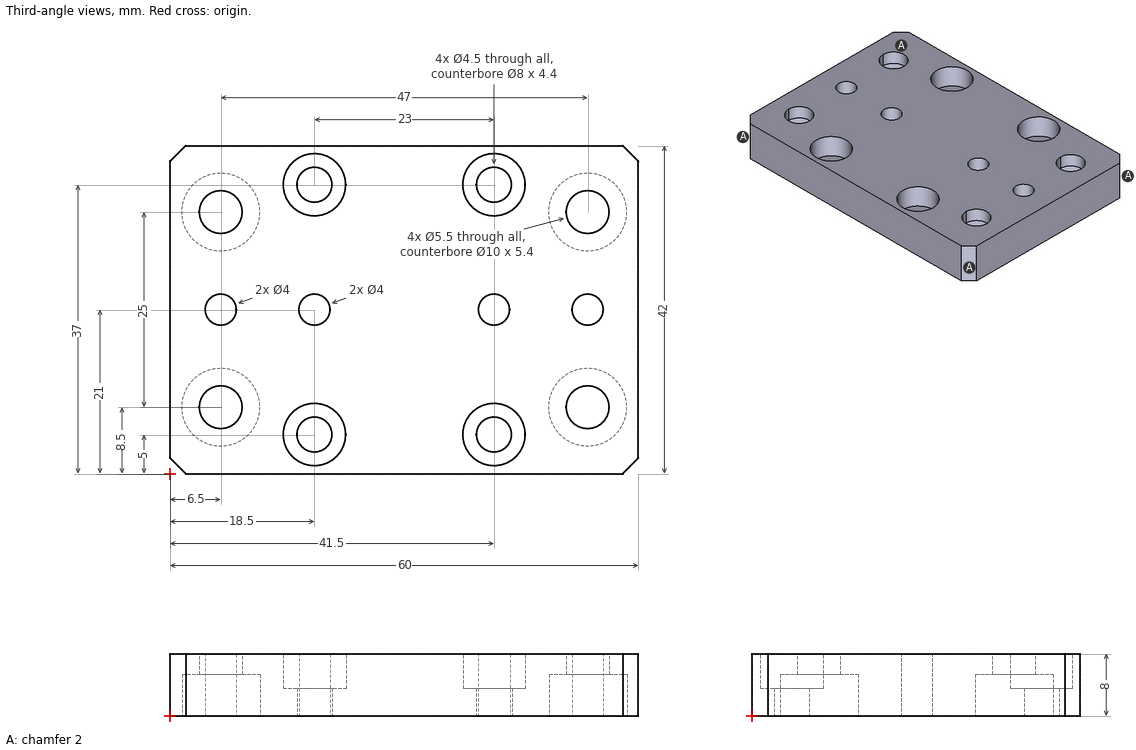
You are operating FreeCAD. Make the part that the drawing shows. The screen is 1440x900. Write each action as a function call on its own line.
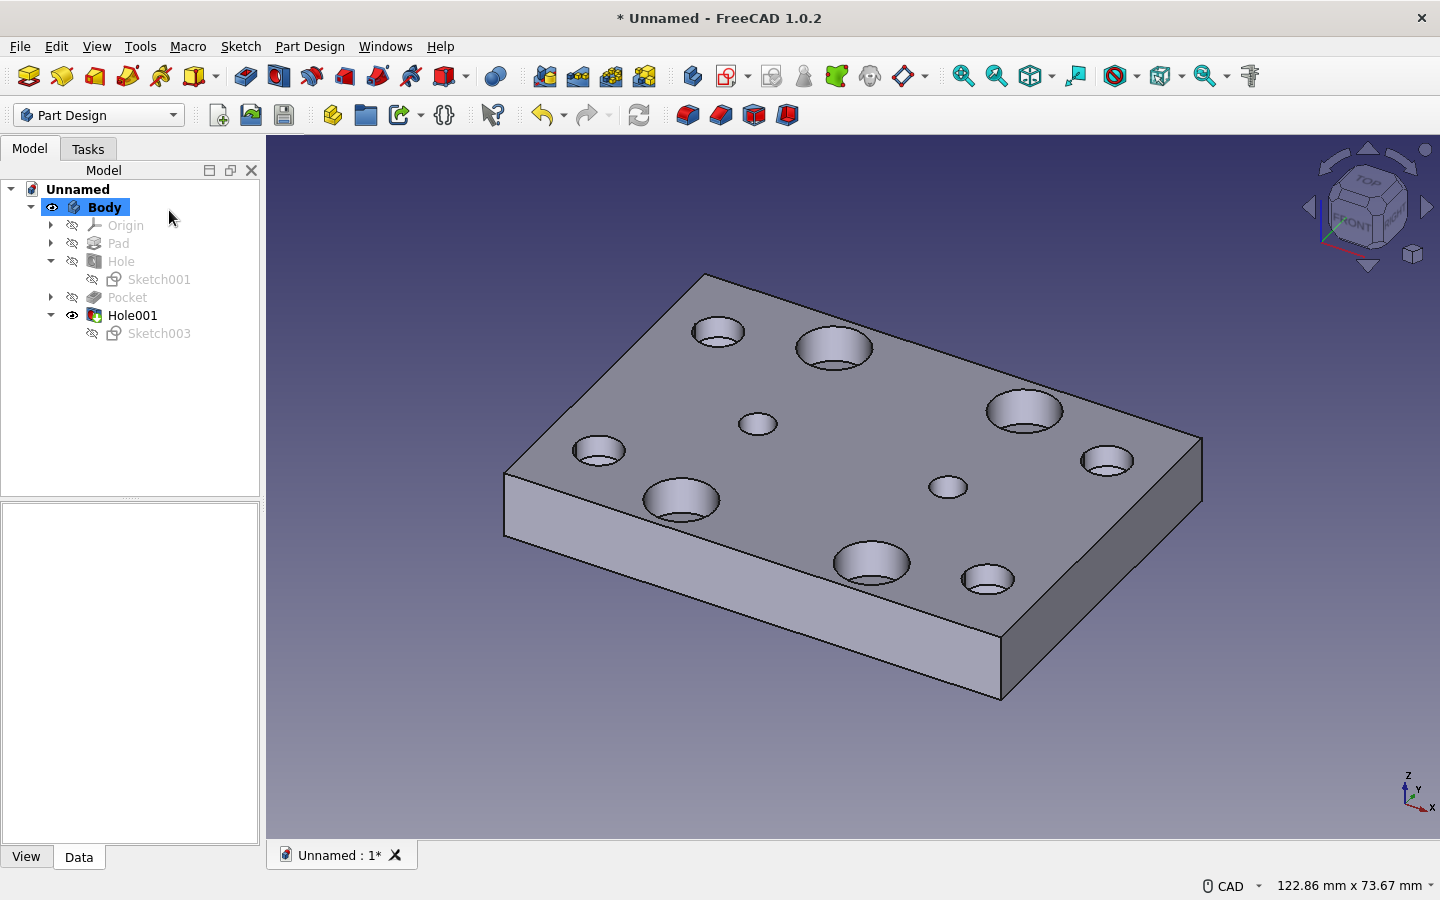
click(882, 426)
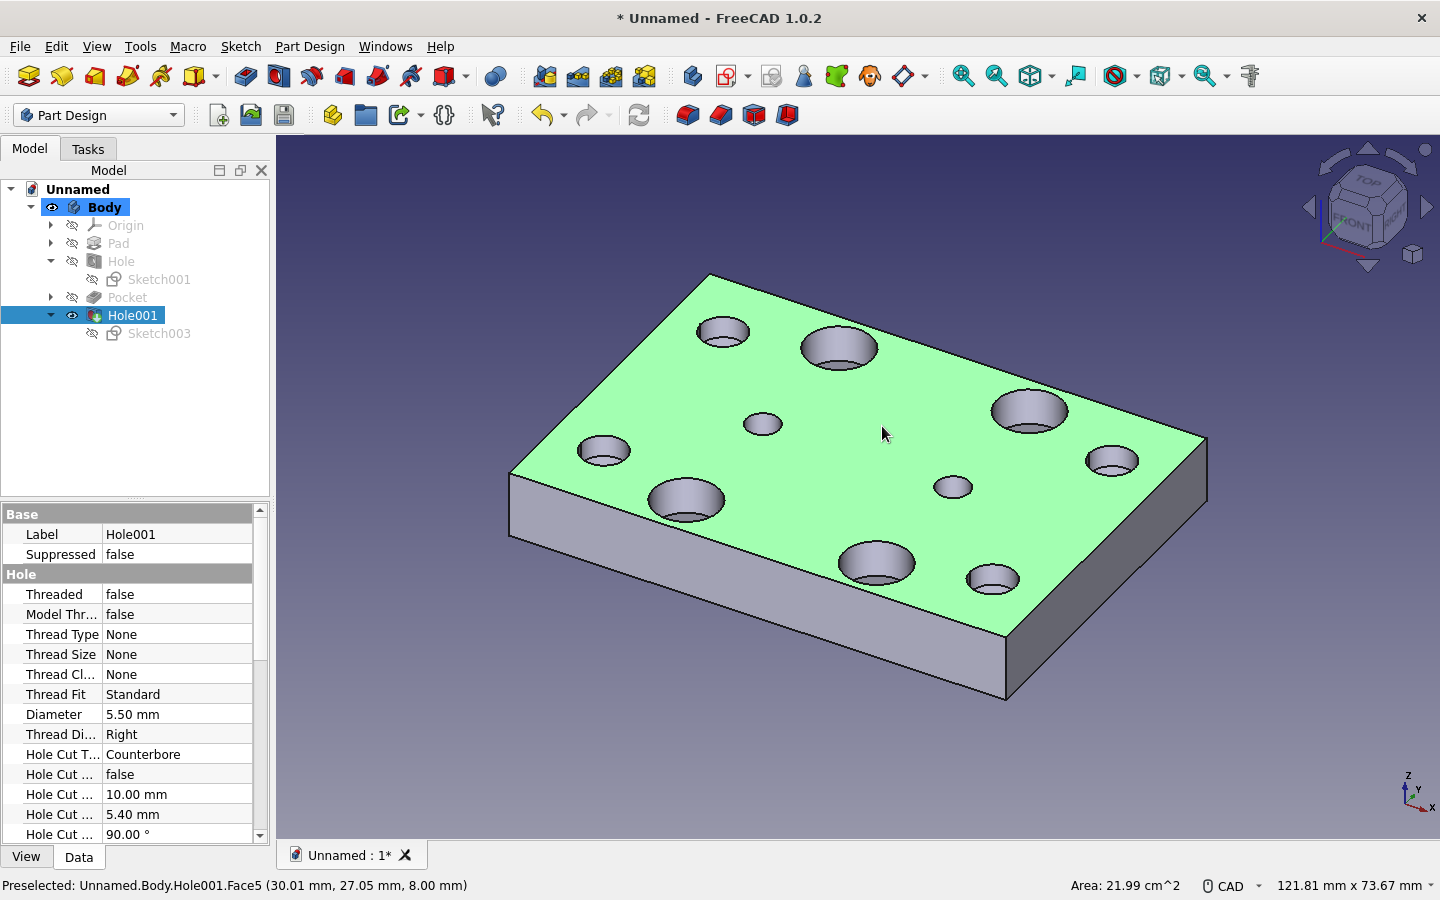
click(726, 76)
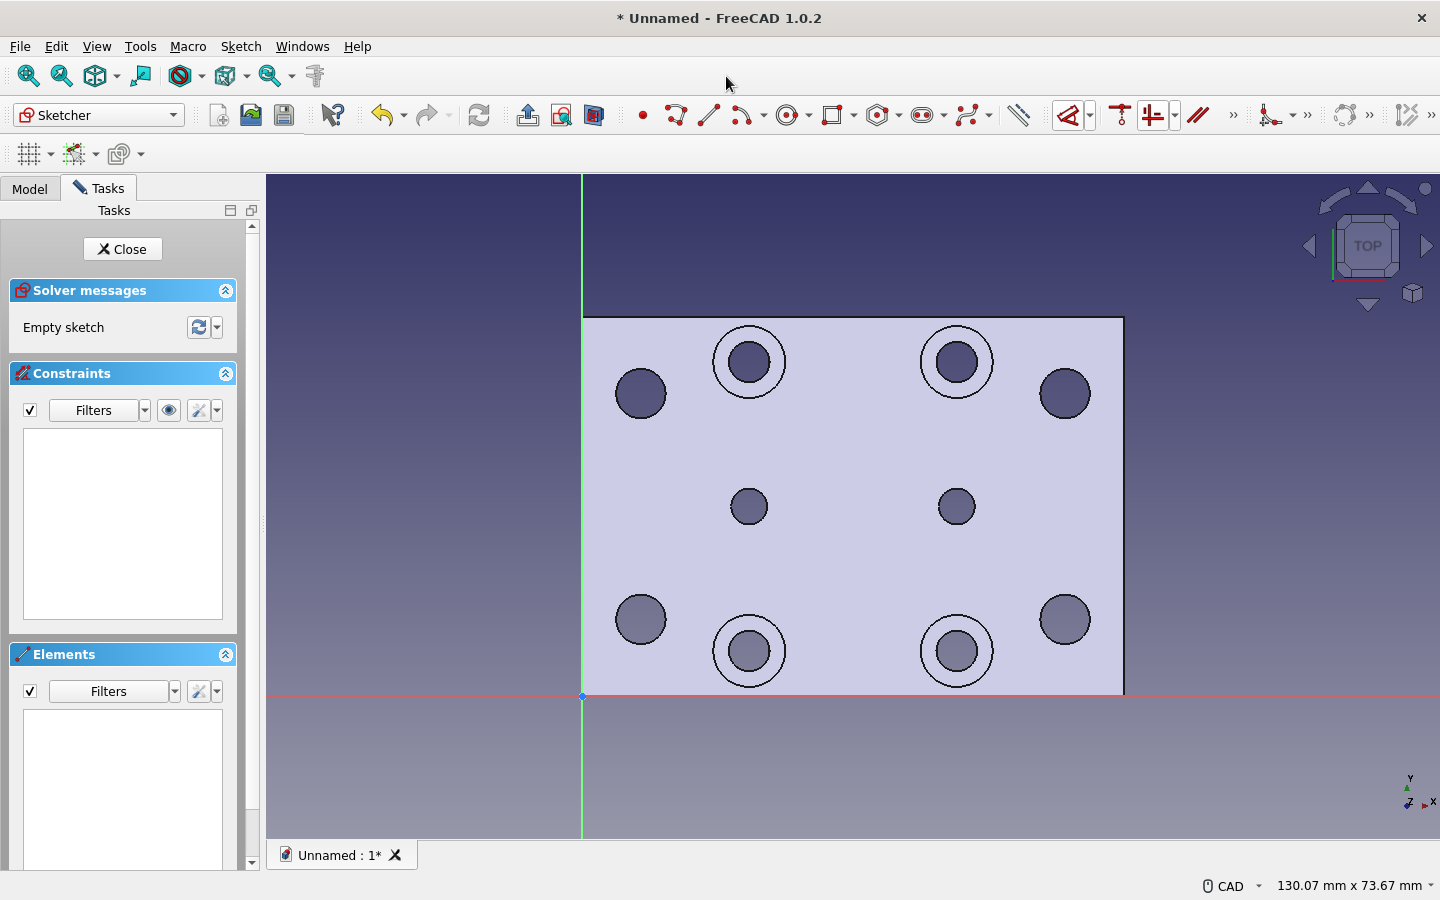
scroll(931, 767, up, 2)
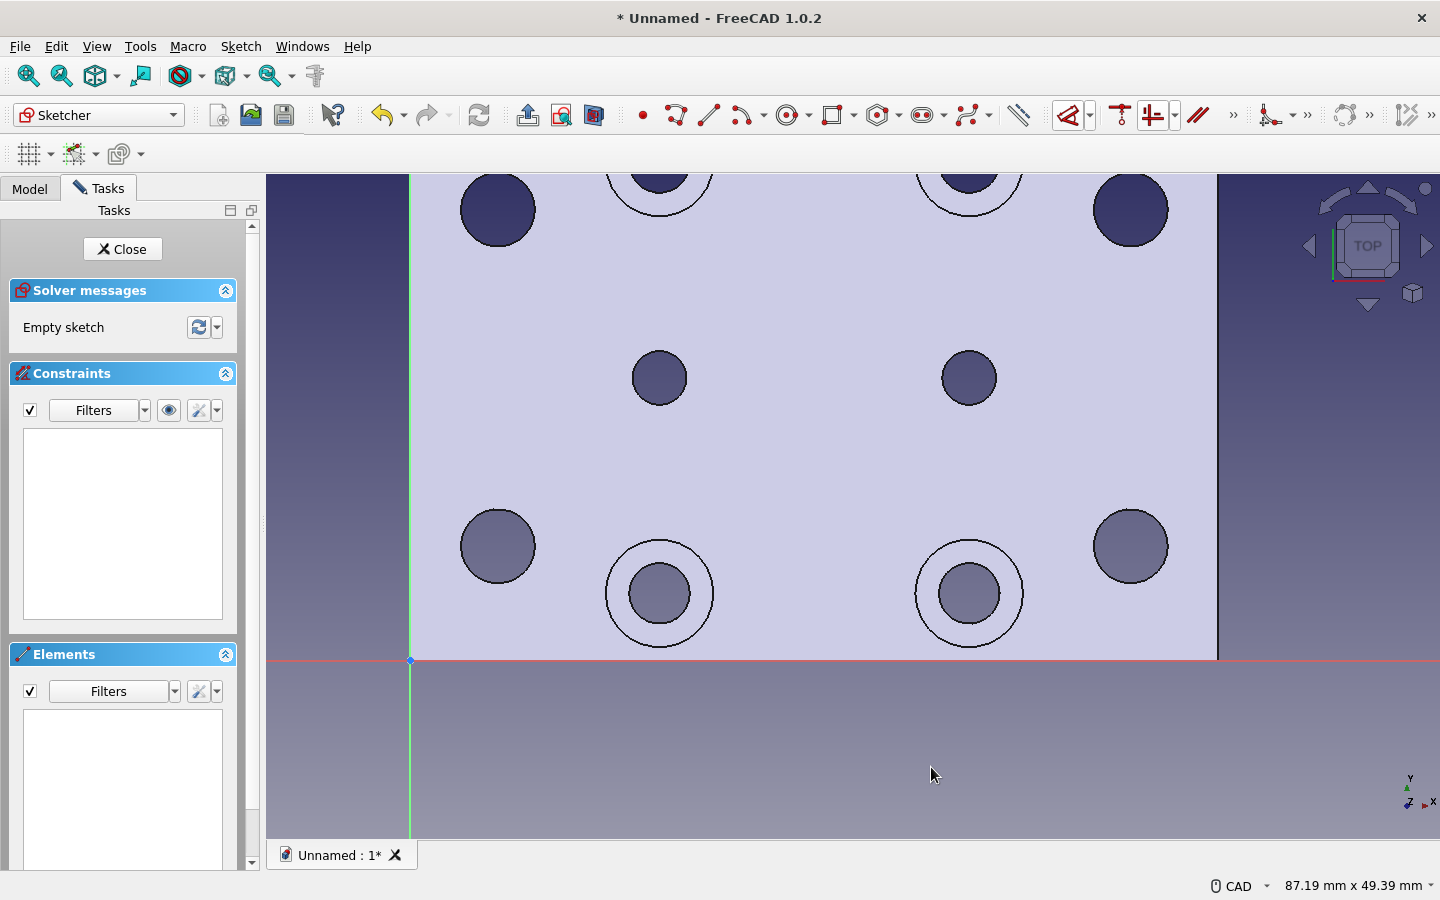
key(g)
key(c)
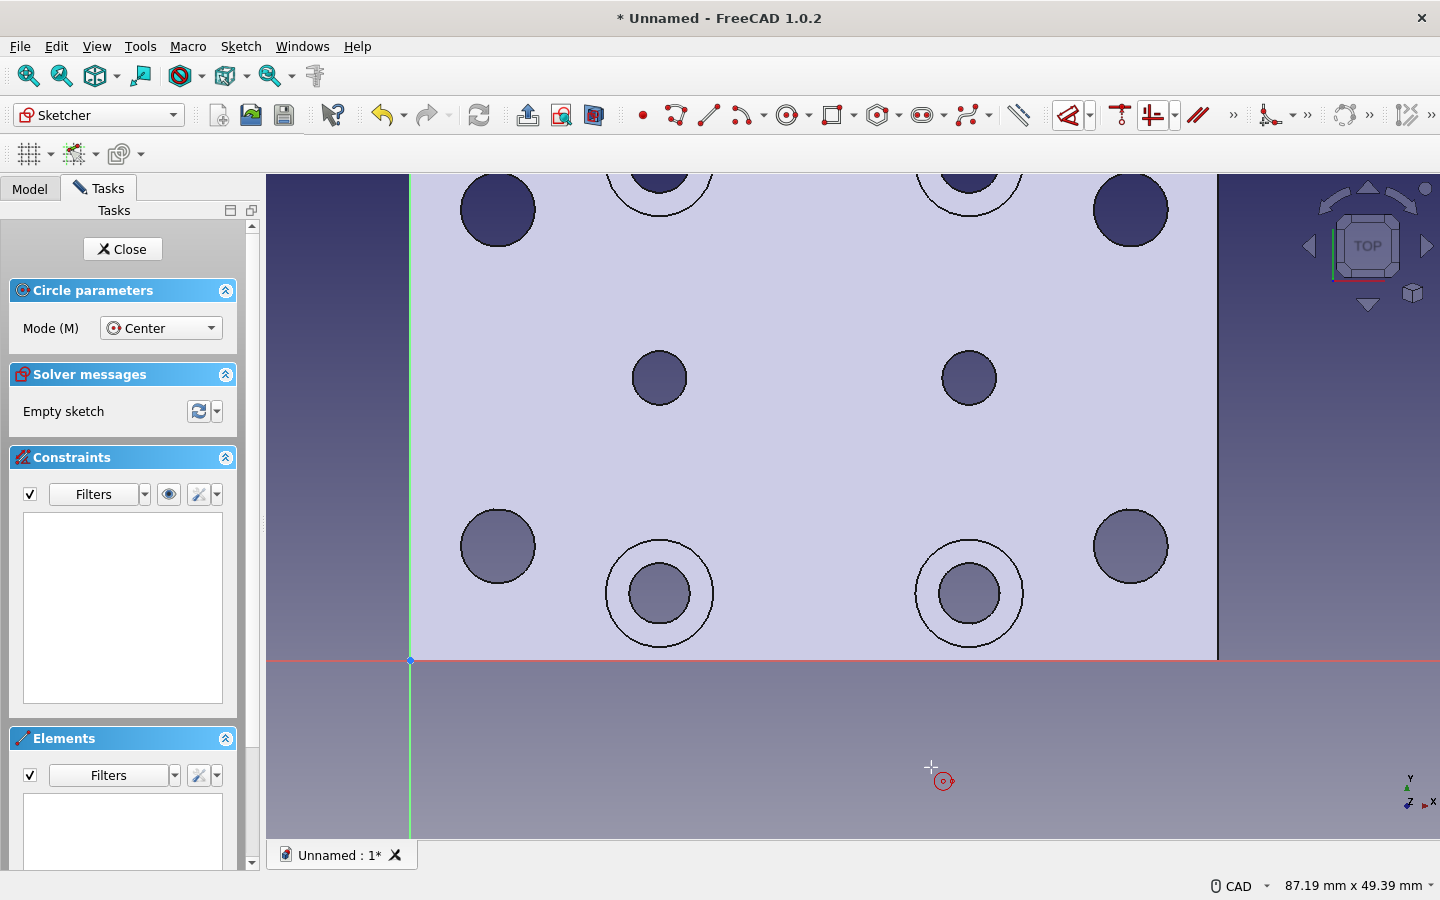
click(498, 378)
click(517, 359)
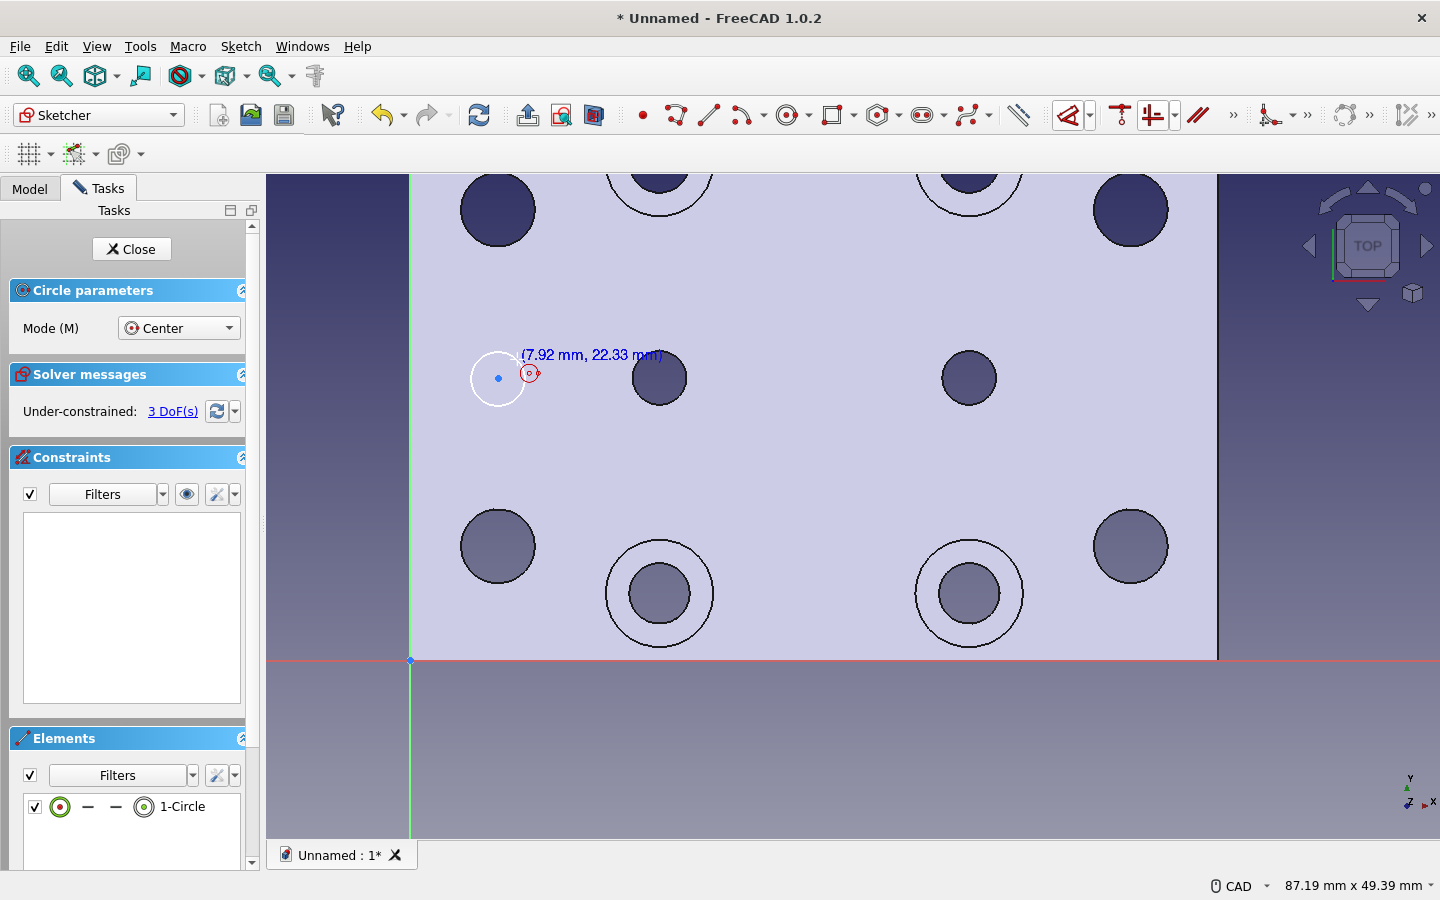
click(1131, 378)
click(1150, 359)
key(Escape)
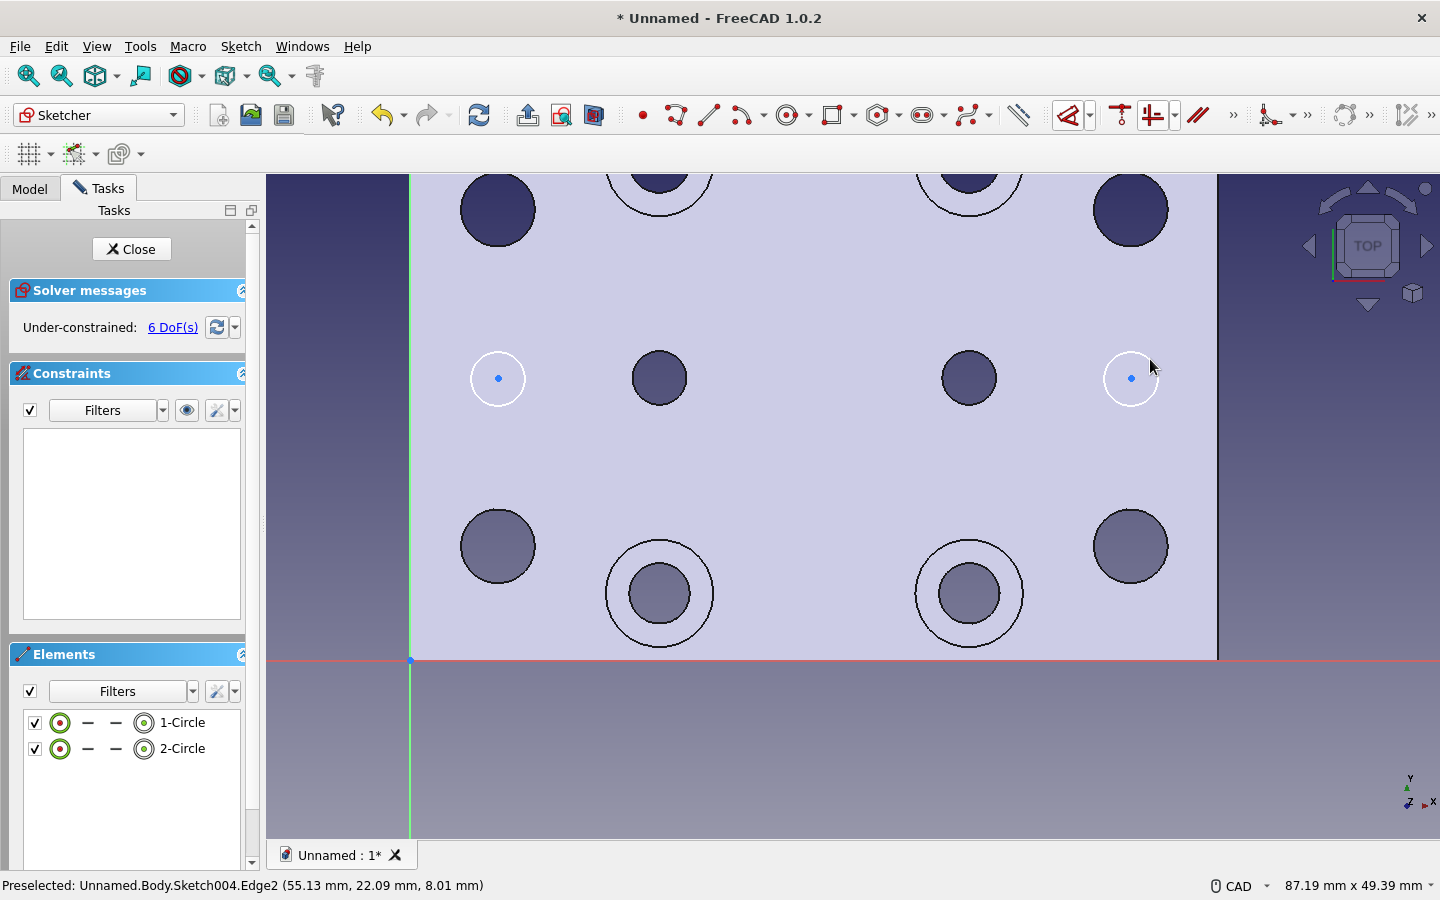
click(517, 360)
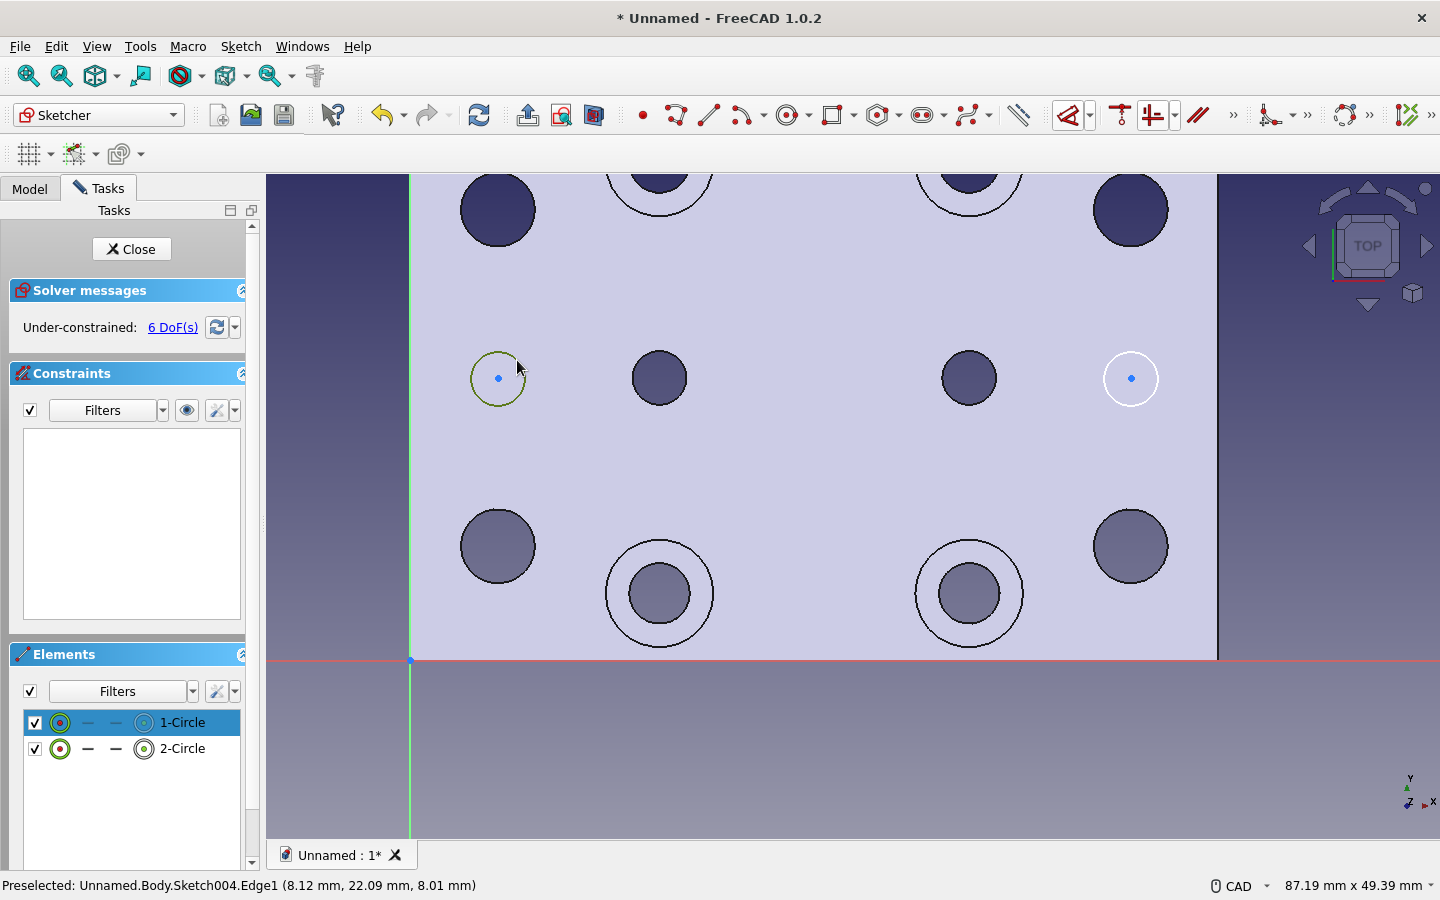
click(1150, 360)